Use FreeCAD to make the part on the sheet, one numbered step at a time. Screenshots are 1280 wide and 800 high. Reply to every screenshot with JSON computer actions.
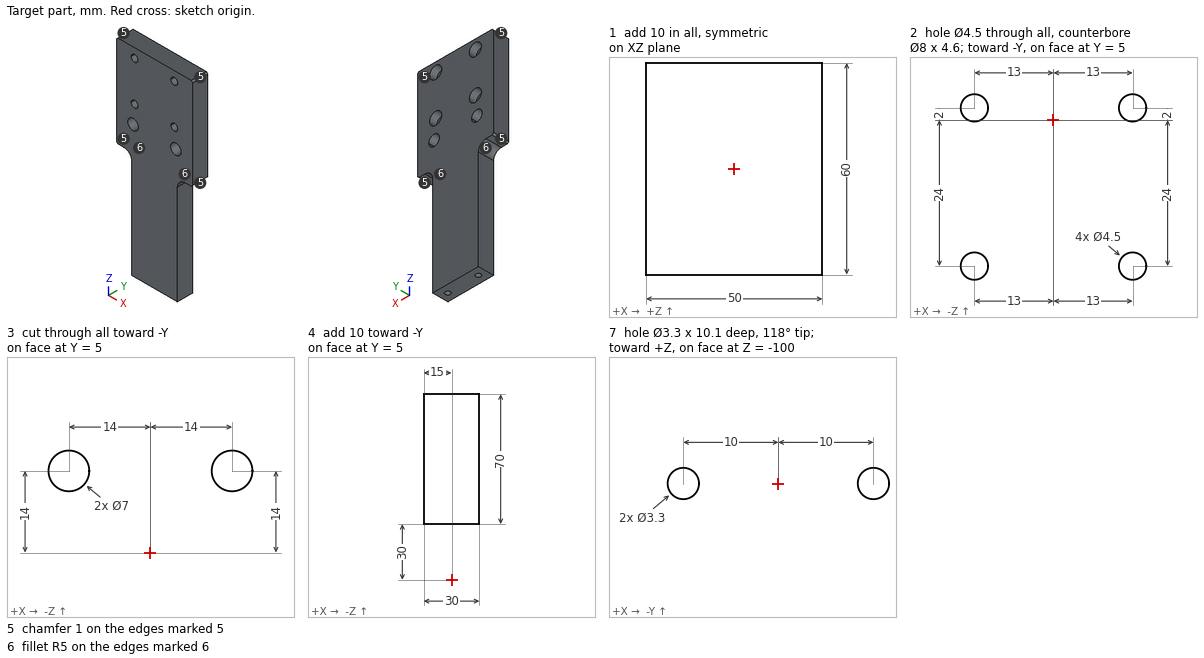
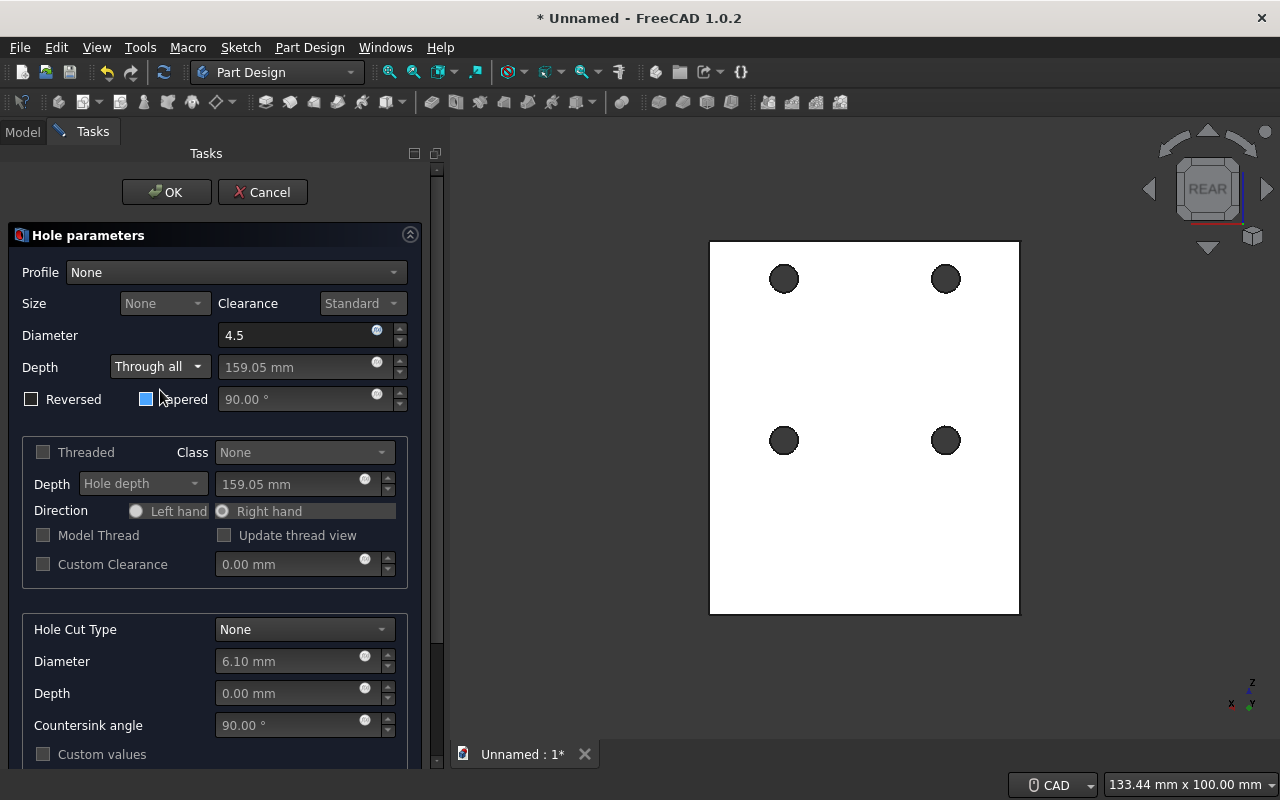
{"action": "left_click", "coordinate": [306, 630]}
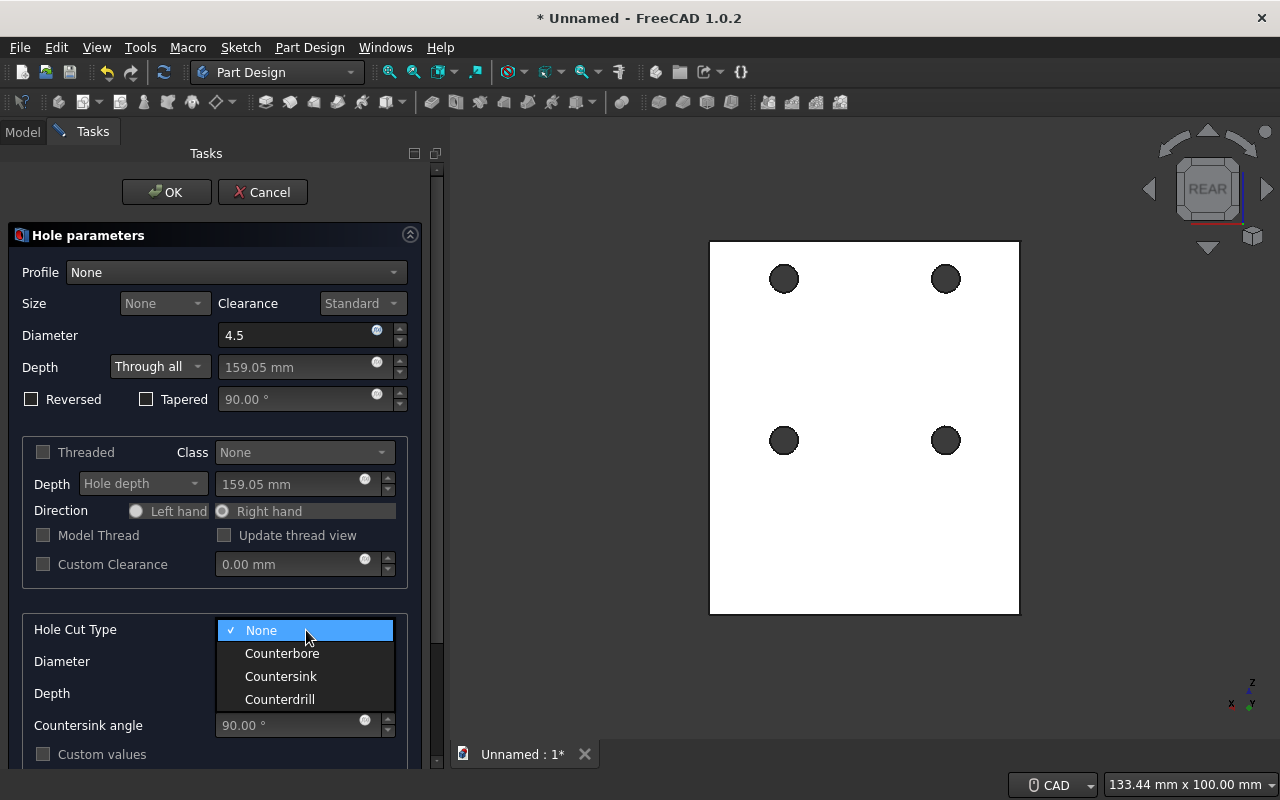
{"action": "left_click", "coordinate": [304, 654]}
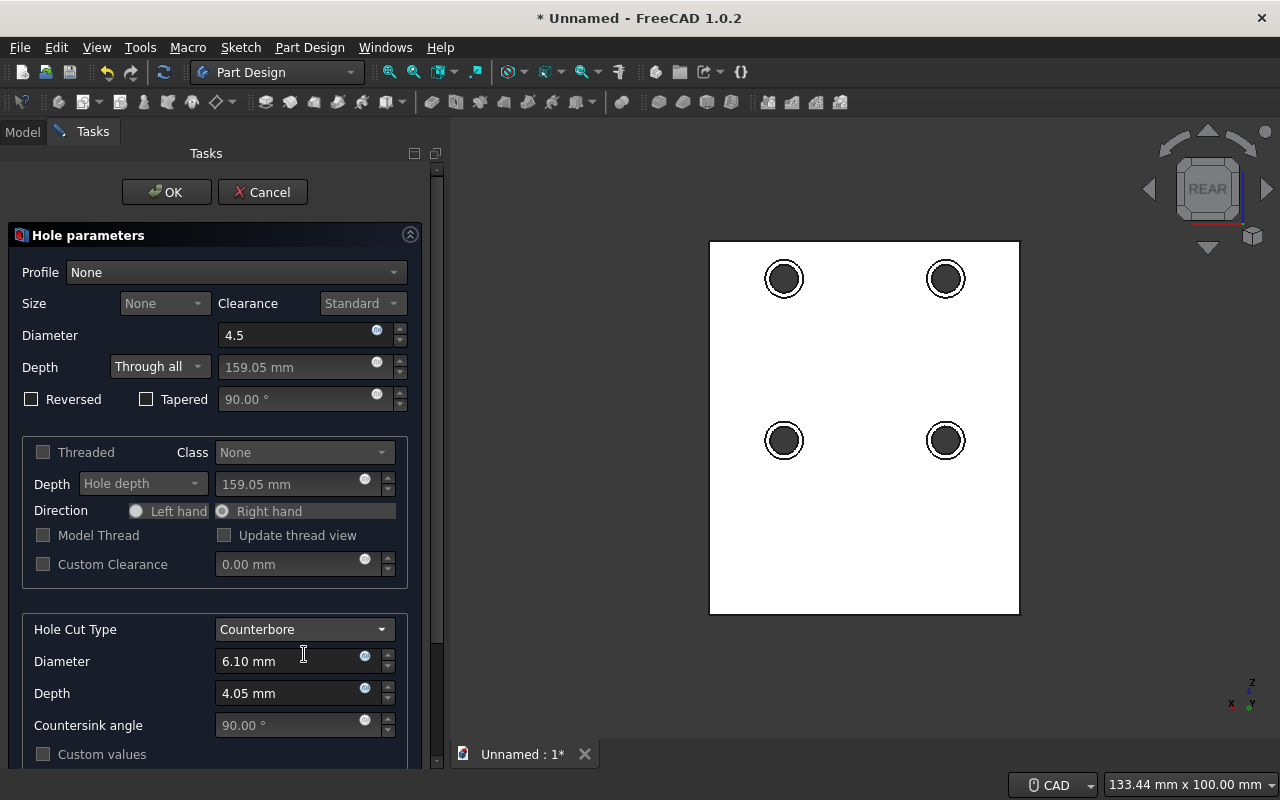
{"action": "triple_click", "coordinate": [298, 661]}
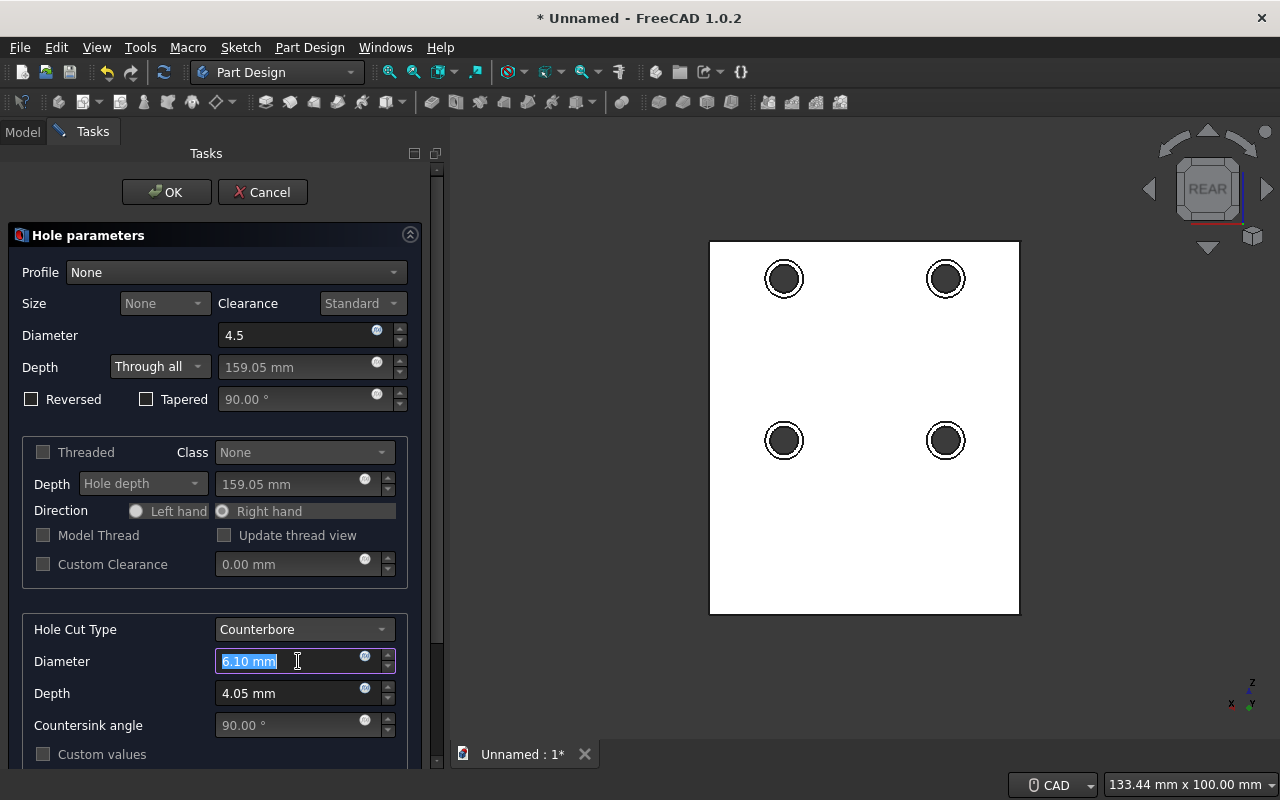
{"action": "type", "text": "8"}
{"action": "key", "text": "Tab"}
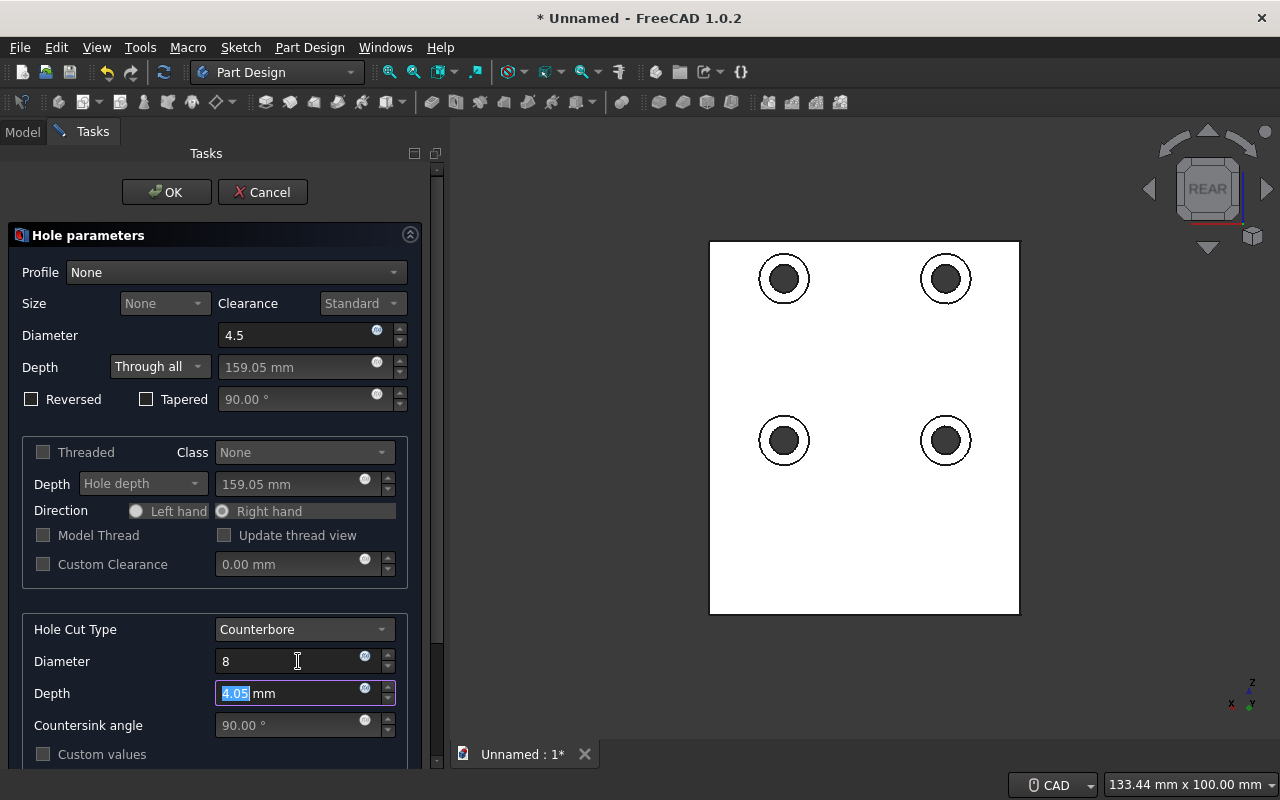
{"action": "type", "text": "4.6"}
{"action": "key", "text": "Tab"}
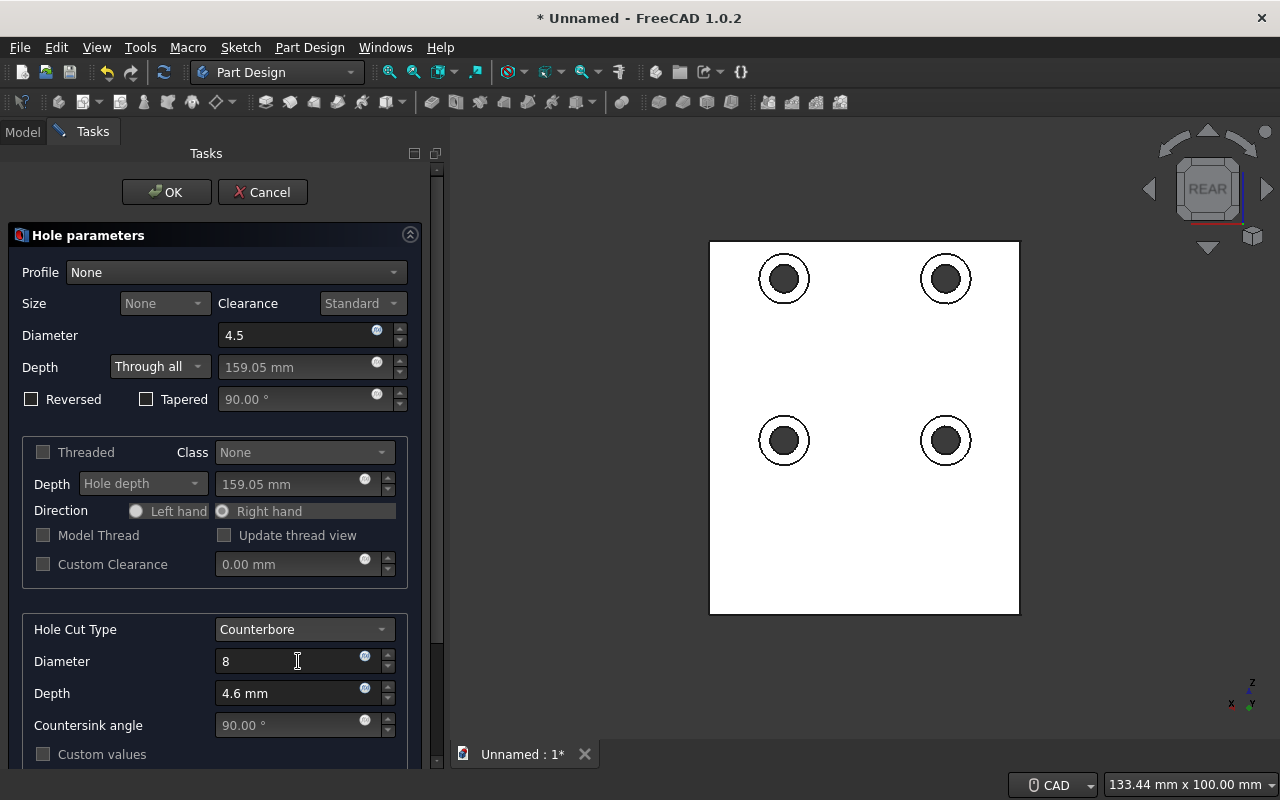
{"action": "left_click", "coordinate": [167, 192]}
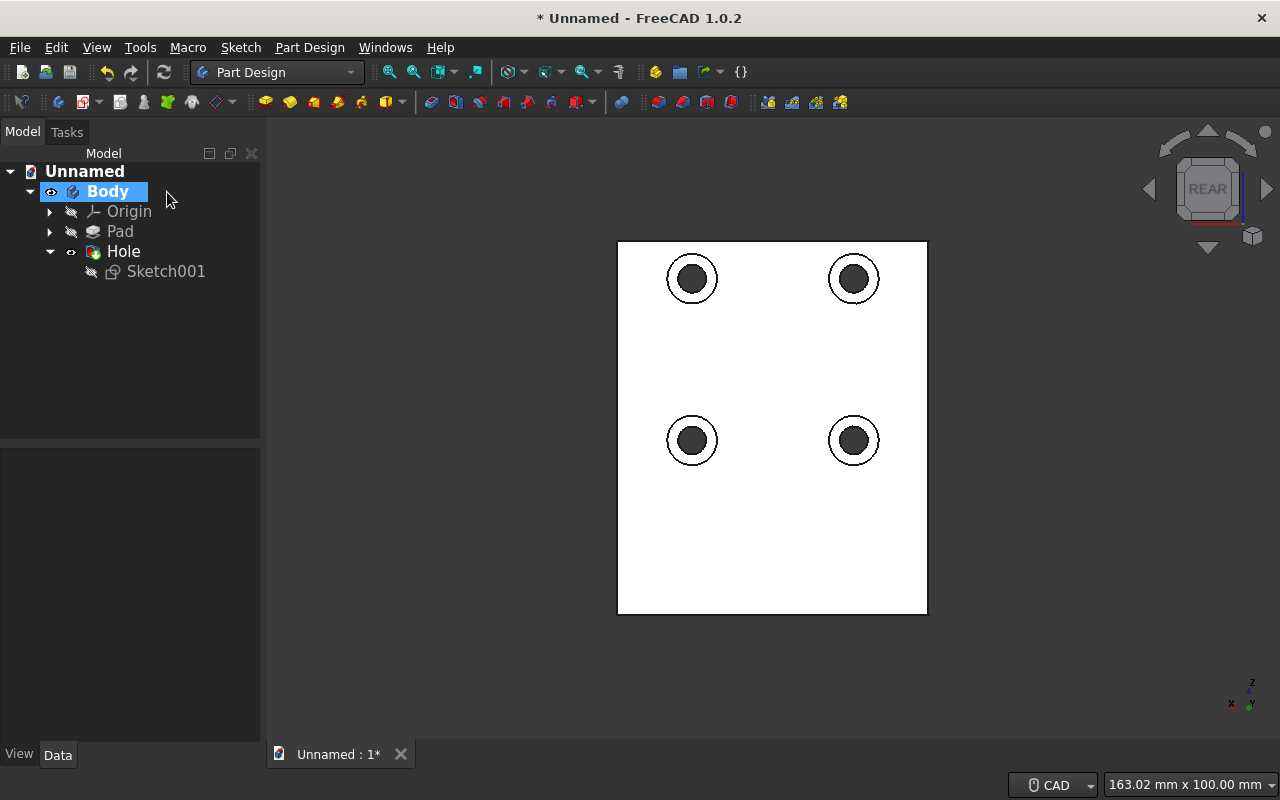
{"action": "left_click", "coordinate": [773, 534]}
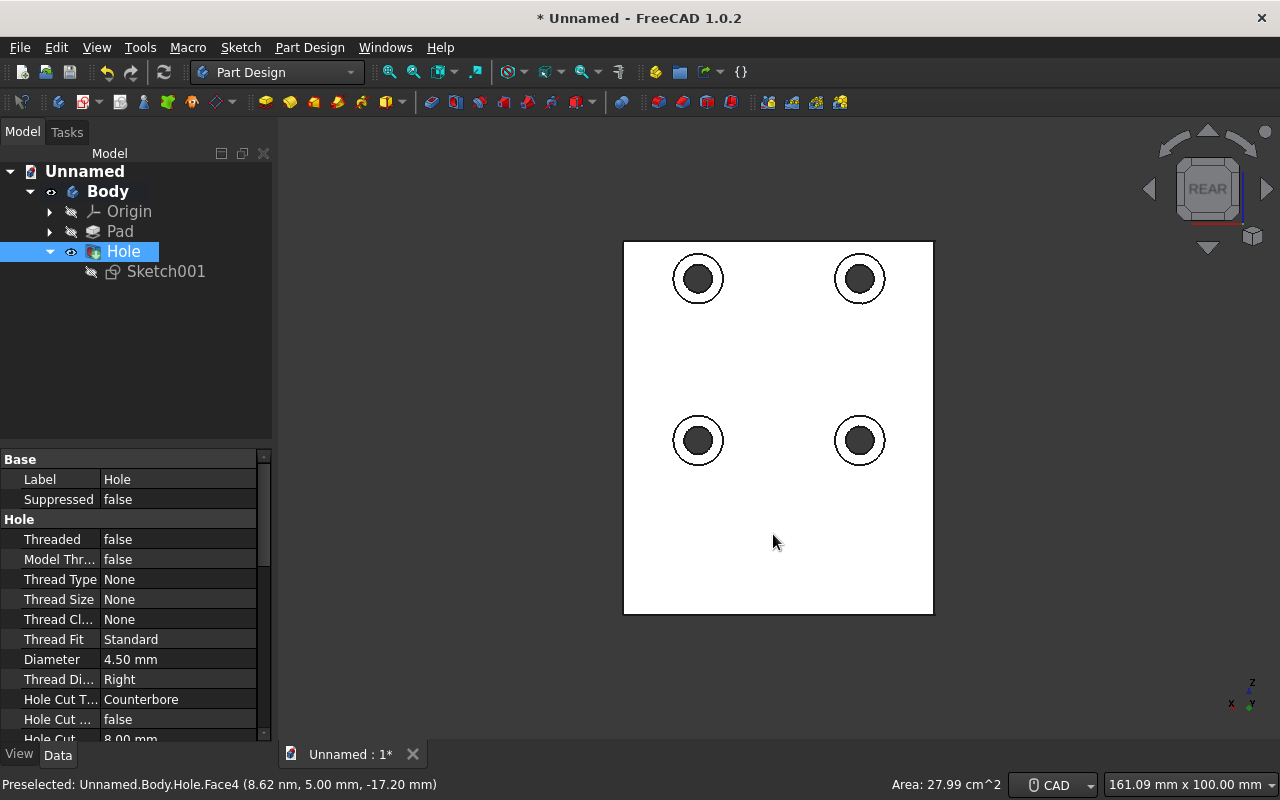
{"action": "left_click", "coordinate": [84, 102]}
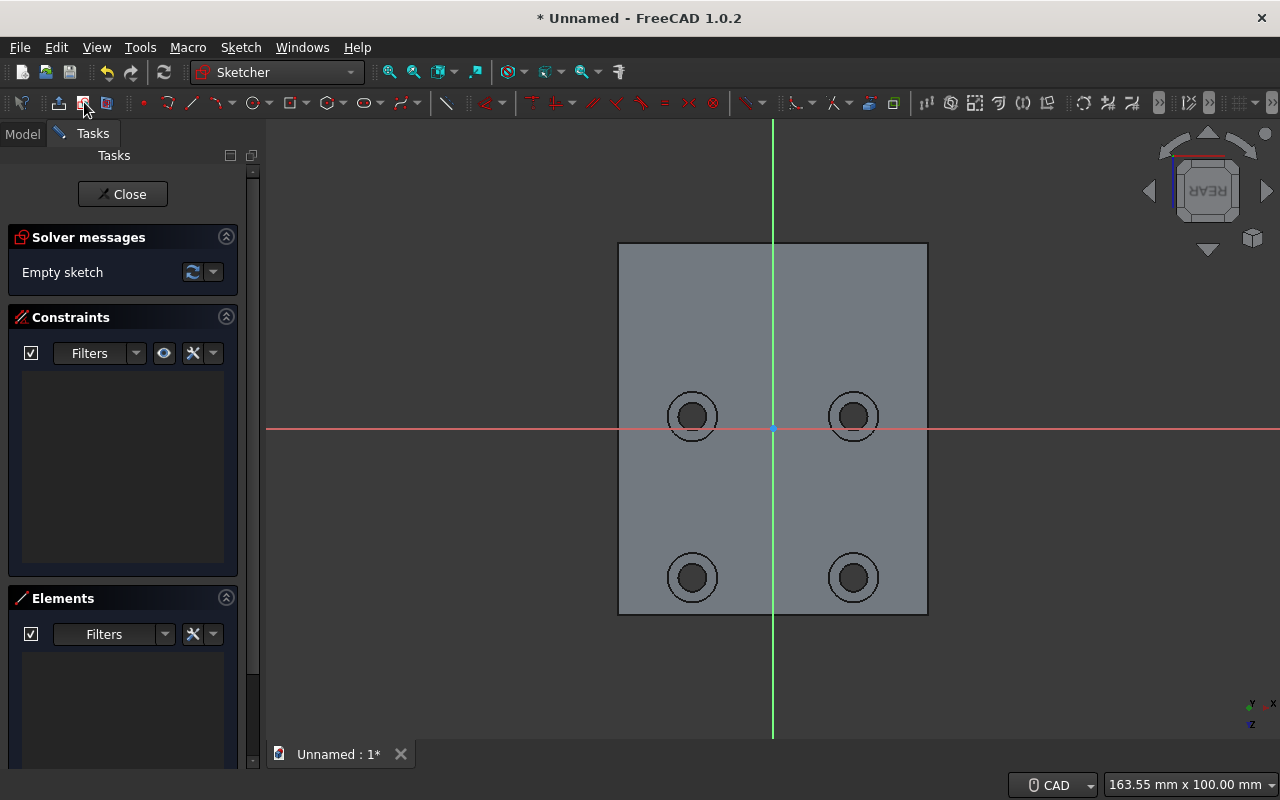
{"action": "scroll", "coordinate": [813, 343], "scroll_direction": "up", "scroll_amount": 5}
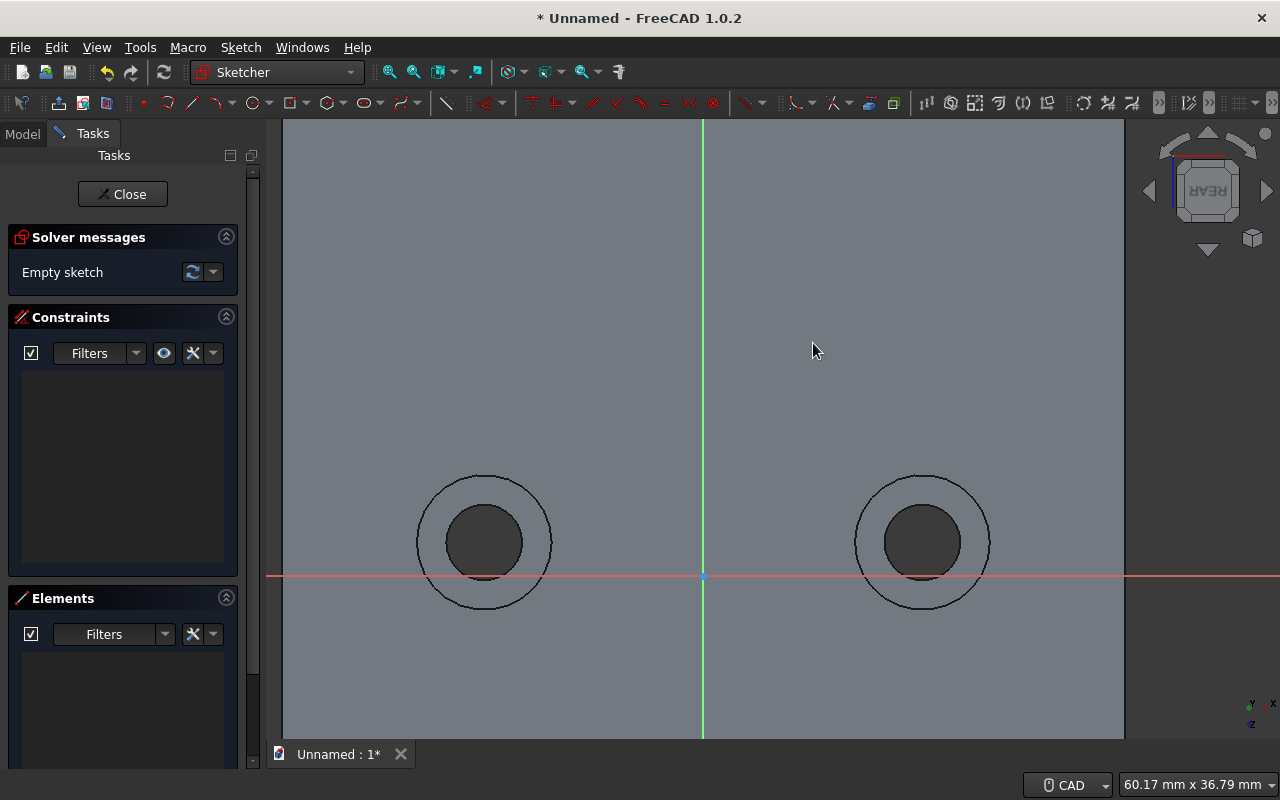
{"action": "left_click", "coordinate": [254, 104]}